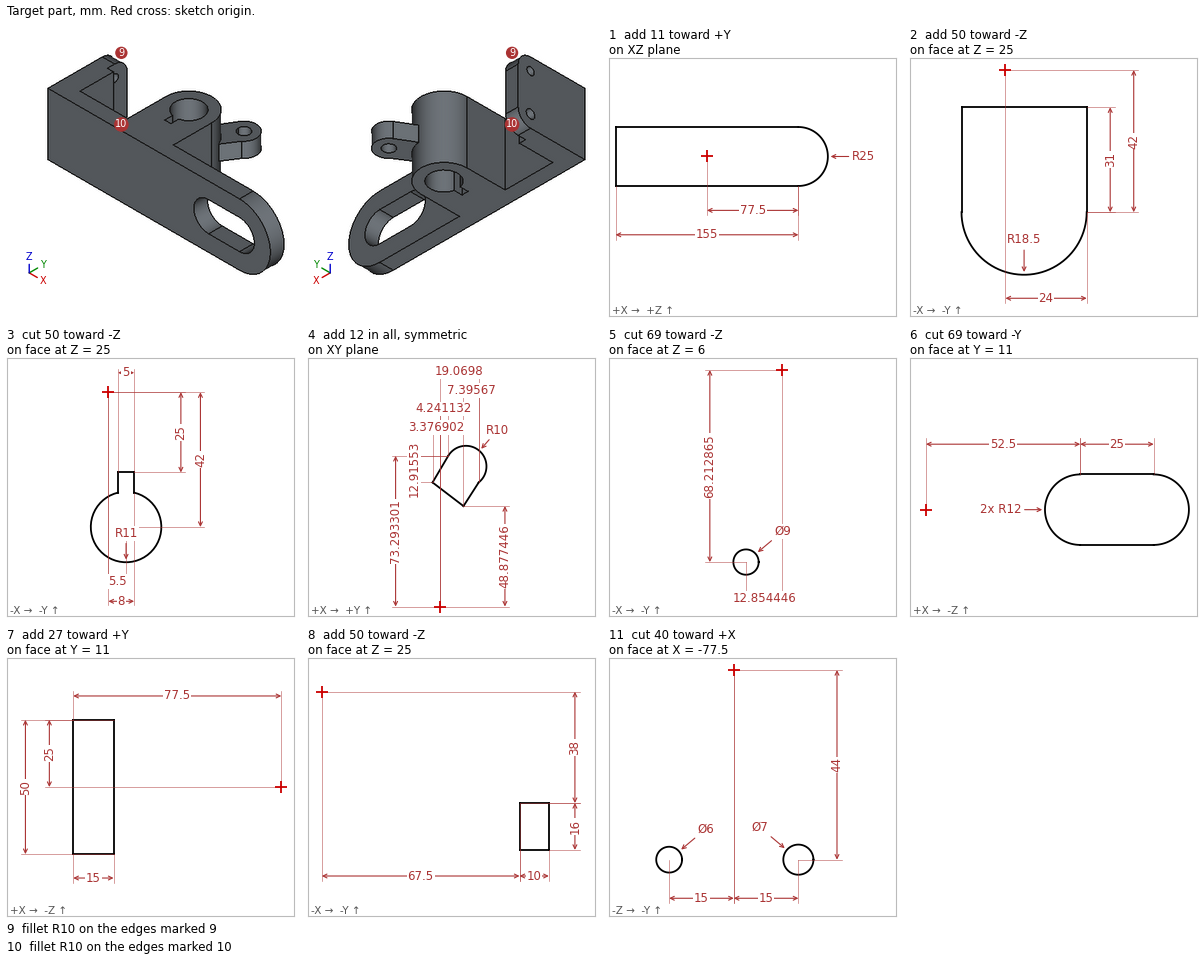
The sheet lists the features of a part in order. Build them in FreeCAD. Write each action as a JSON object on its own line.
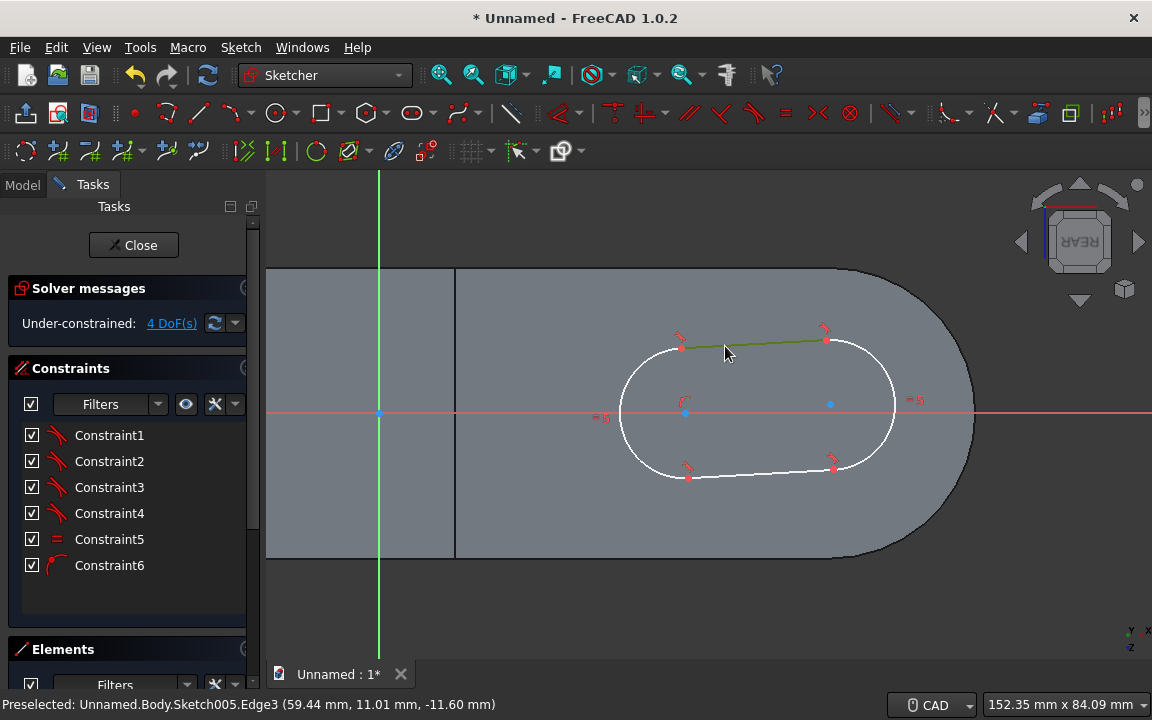
{"action": "key", "text": "h"}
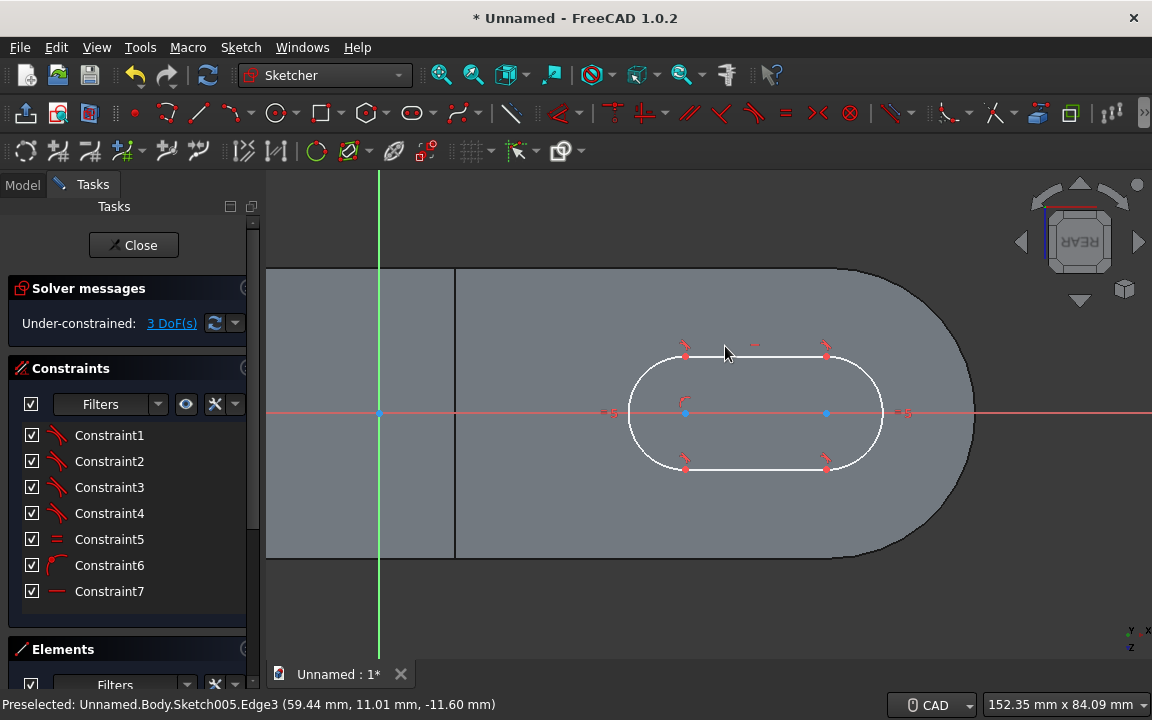
{"action": "left_click", "coordinate": [558, 114]}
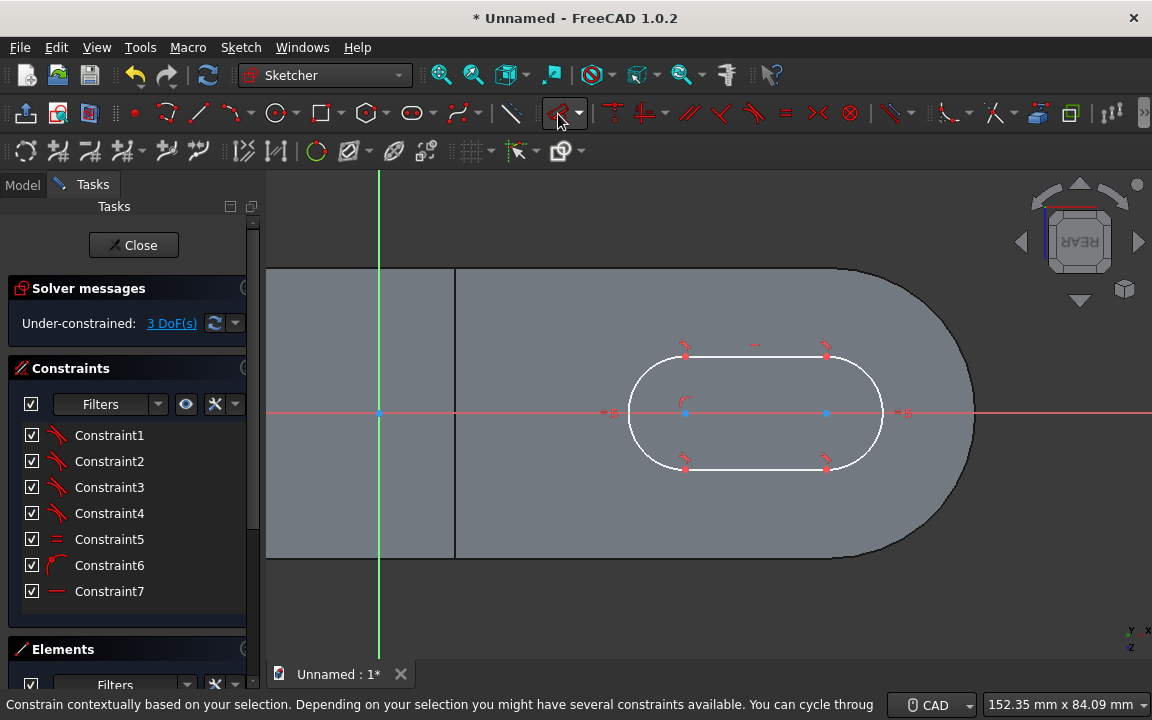
{"action": "left_click", "coordinate": [639, 380]}
{"action": "left_click", "coordinate": [613, 361]}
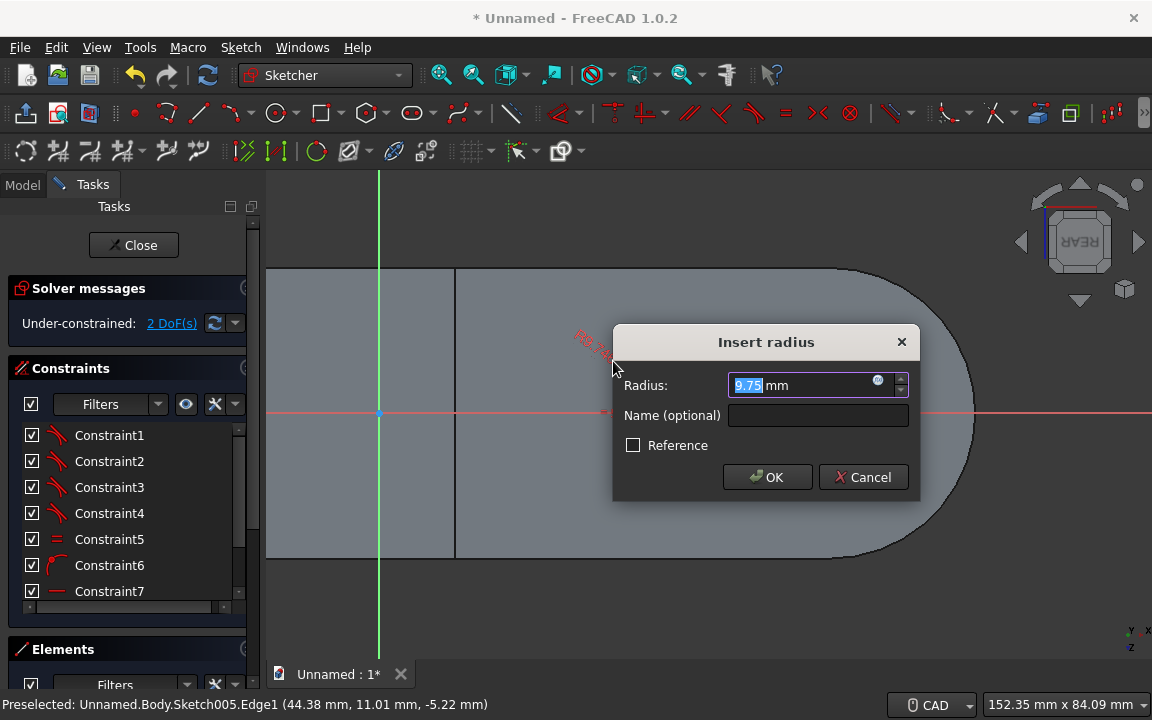
{"action": "type", "text": "12"}
{"action": "key", "text": "Return"}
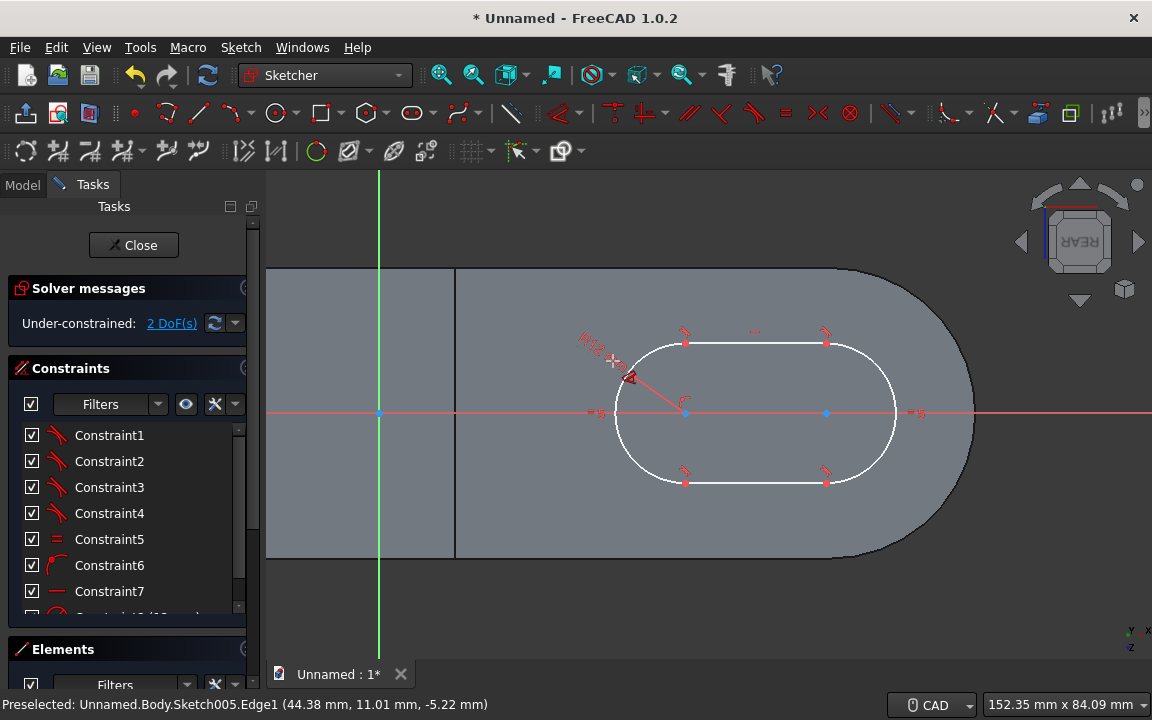
{"action": "left_click", "coordinate": [727, 343]}
{"action": "left_click", "coordinate": [756, 309]}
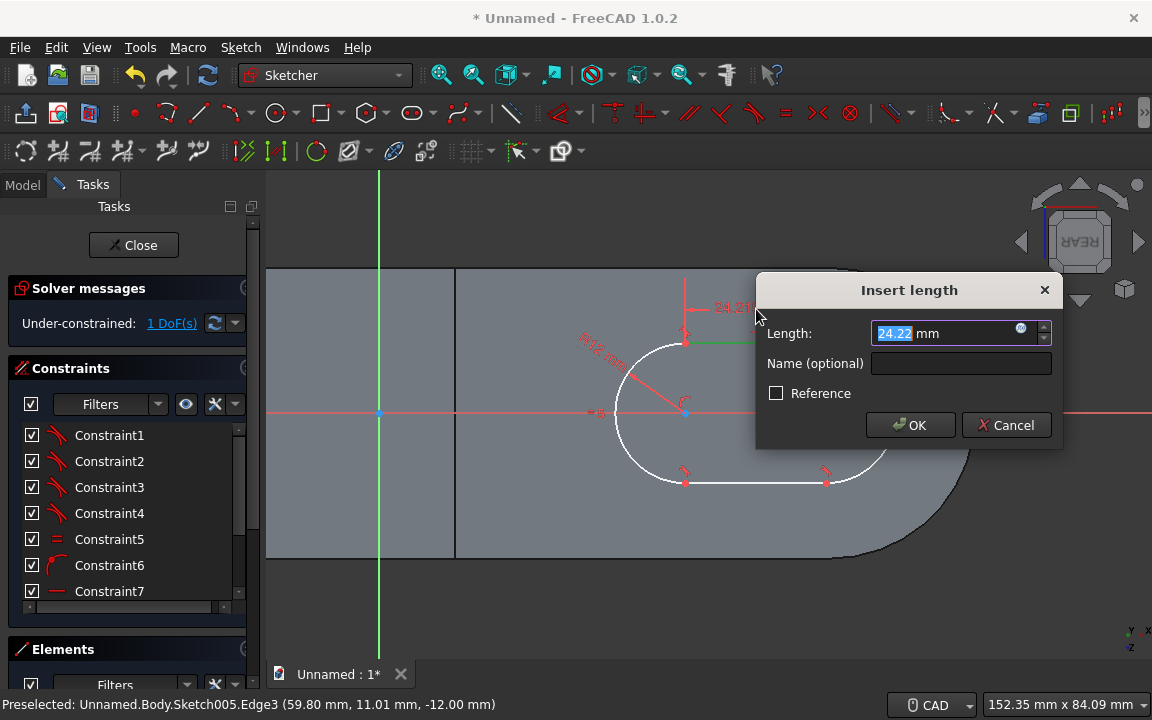
{"action": "type", "text": "25"}
{"action": "key", "text": "Return"}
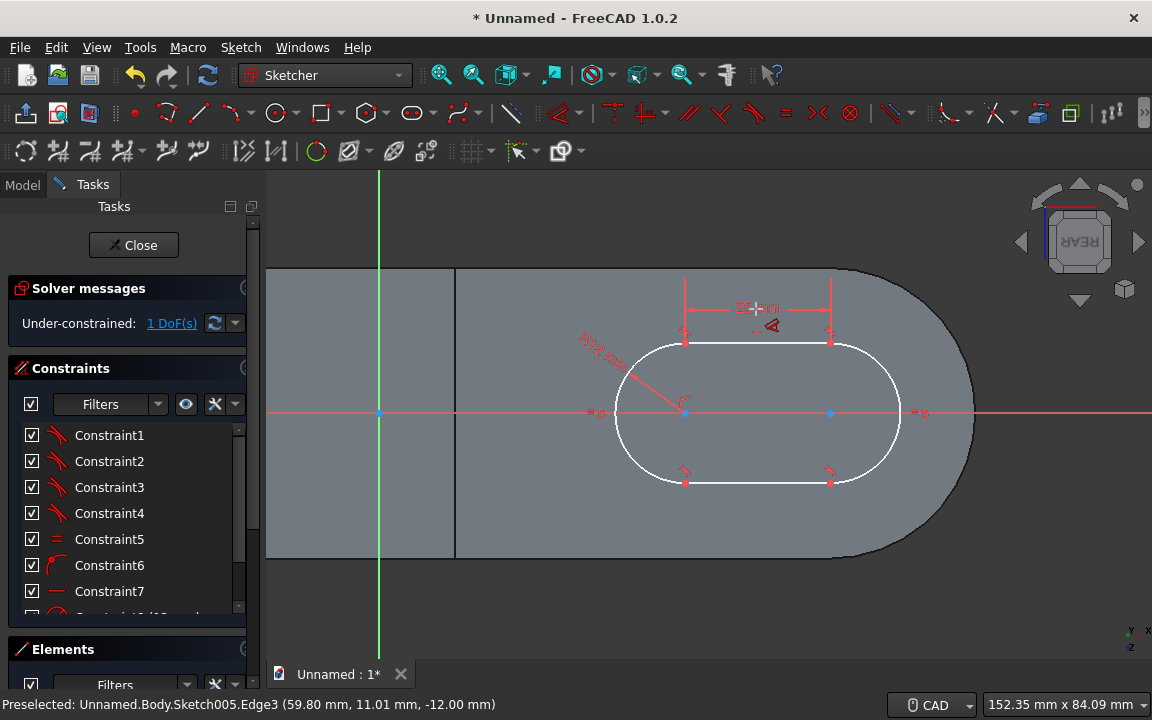
{"action": "left_click", "coordinate": [685, 343]}
{"action": "left_click", "coordinate": [532, 309]}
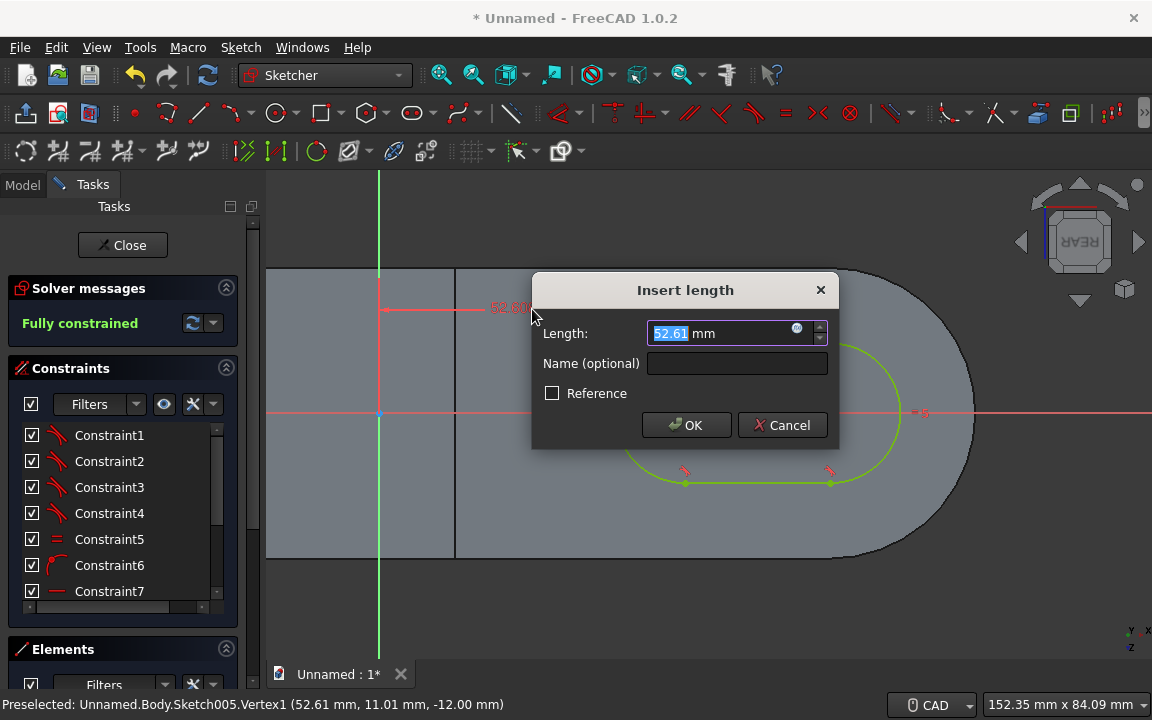
{"action": "type", "text": "52.5"}
{"action": "key", "text": "Return"}
{"action": "key", "text": "Escape"}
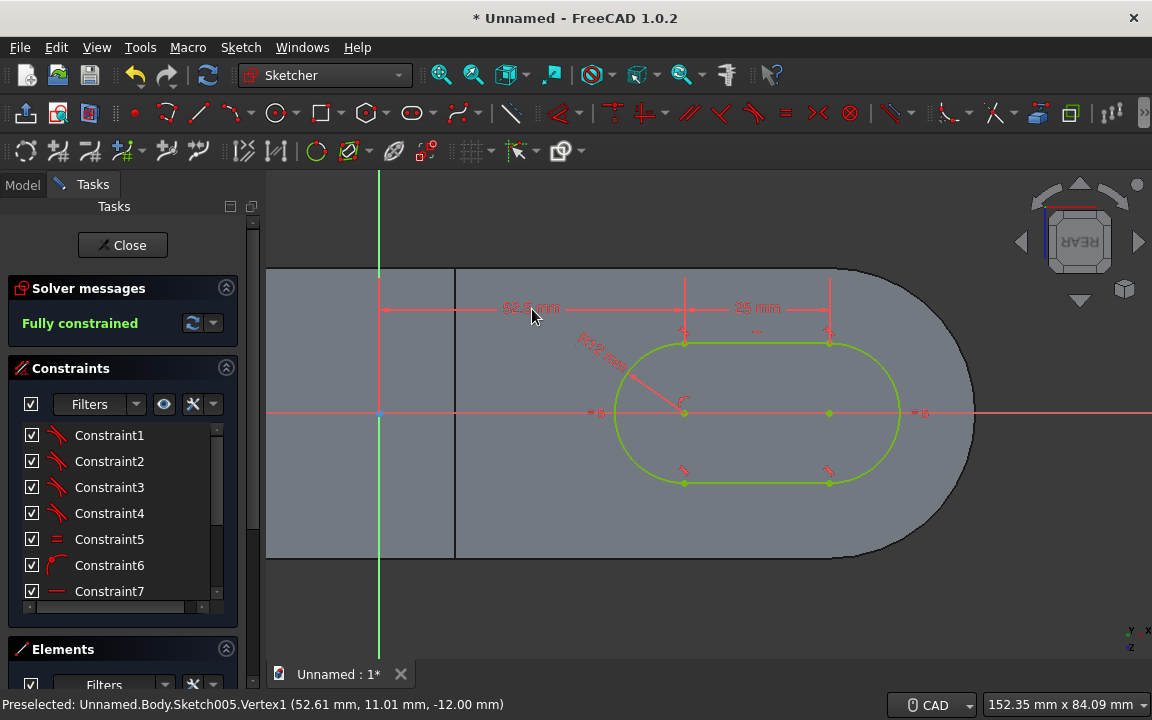
{"action": "left_click", "coordinate": [123, 245]}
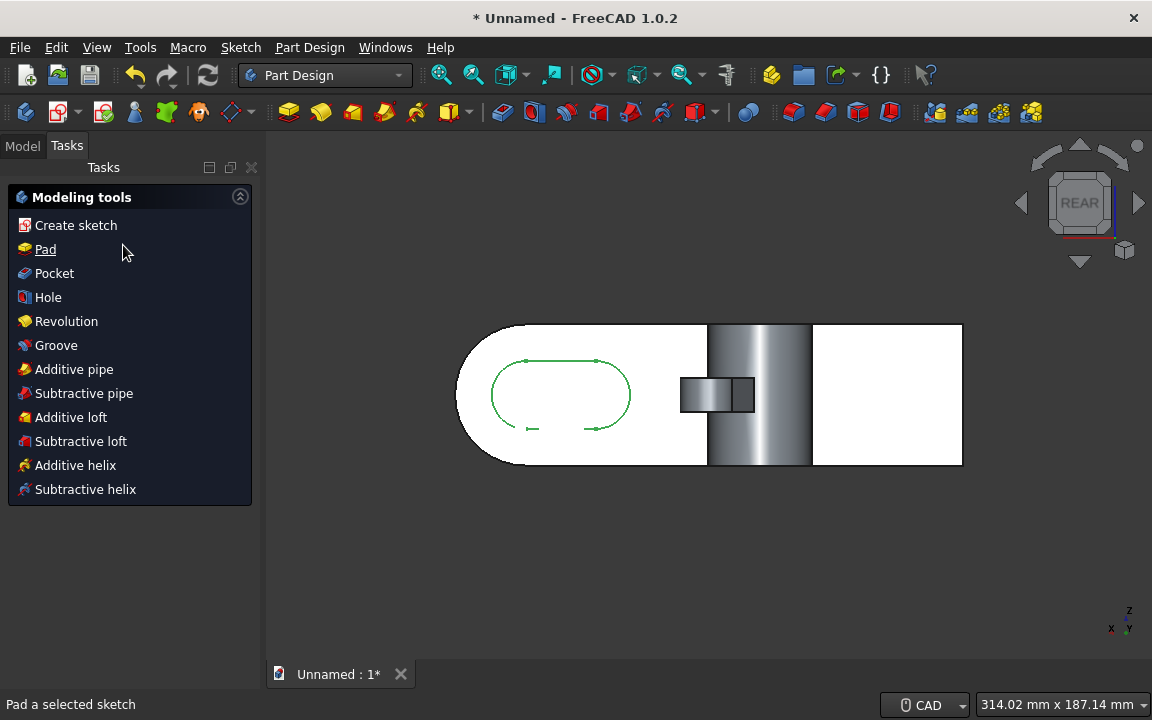
{"action": "left_click", "coordinate": [504, 112]}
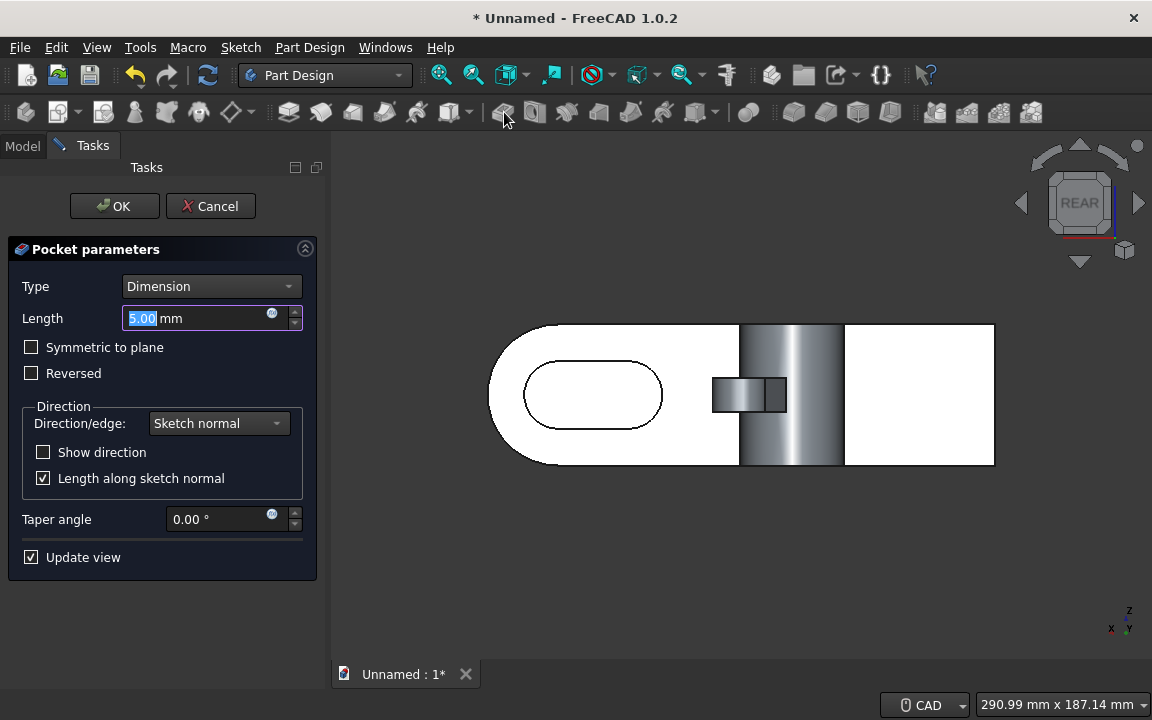
{"action": "type", "text": "69"}
{"action": "key", "text": "Tab"}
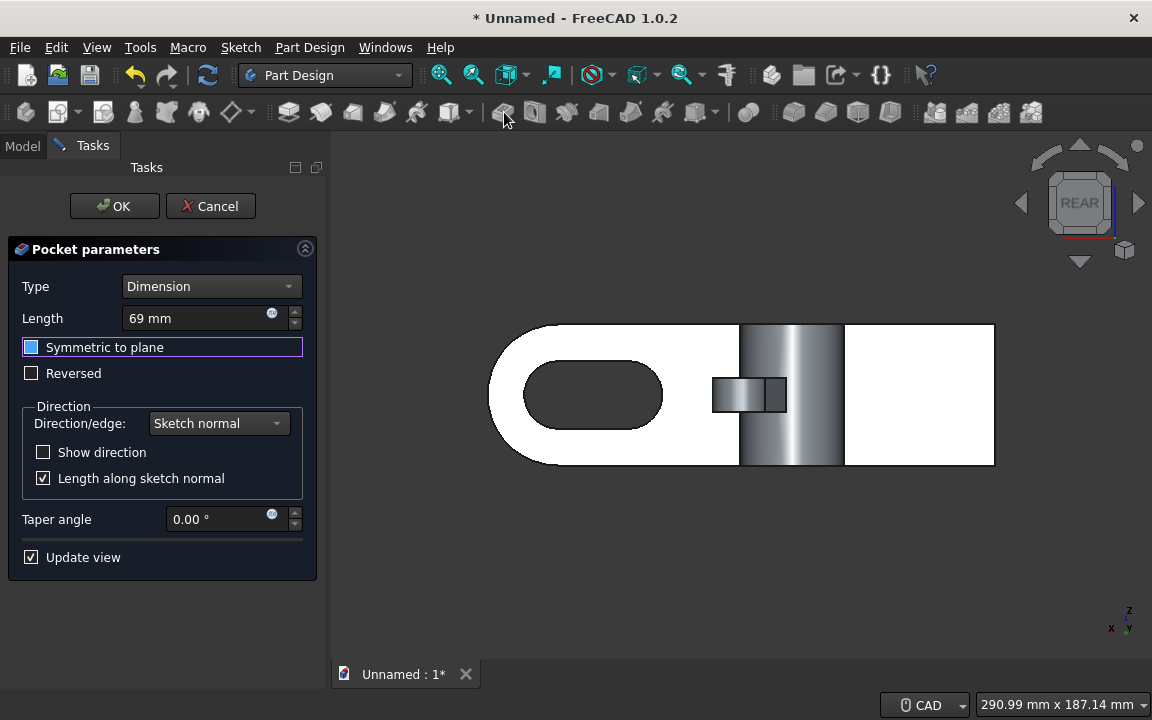
{"action": "left_click", "coordinate": [115, 206]}